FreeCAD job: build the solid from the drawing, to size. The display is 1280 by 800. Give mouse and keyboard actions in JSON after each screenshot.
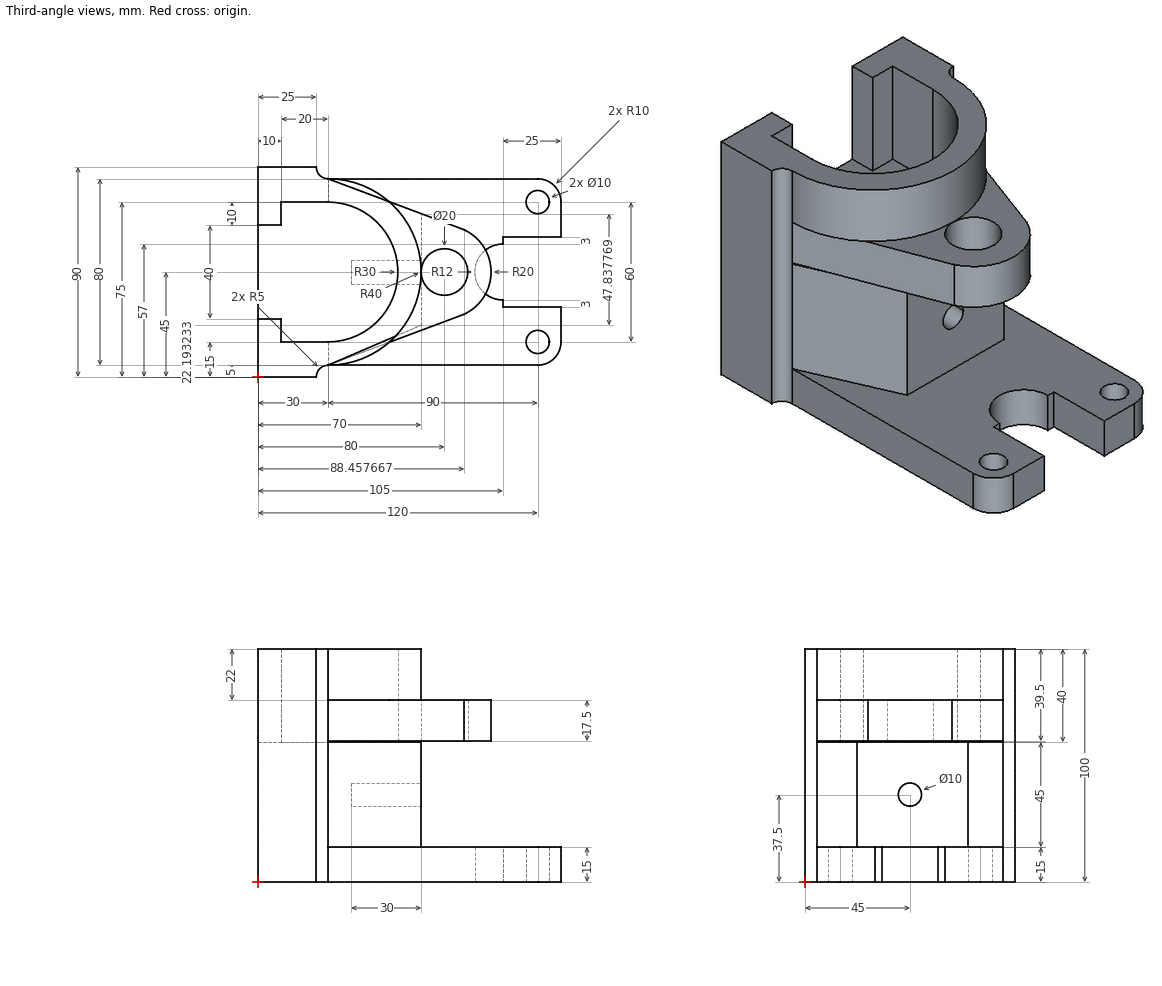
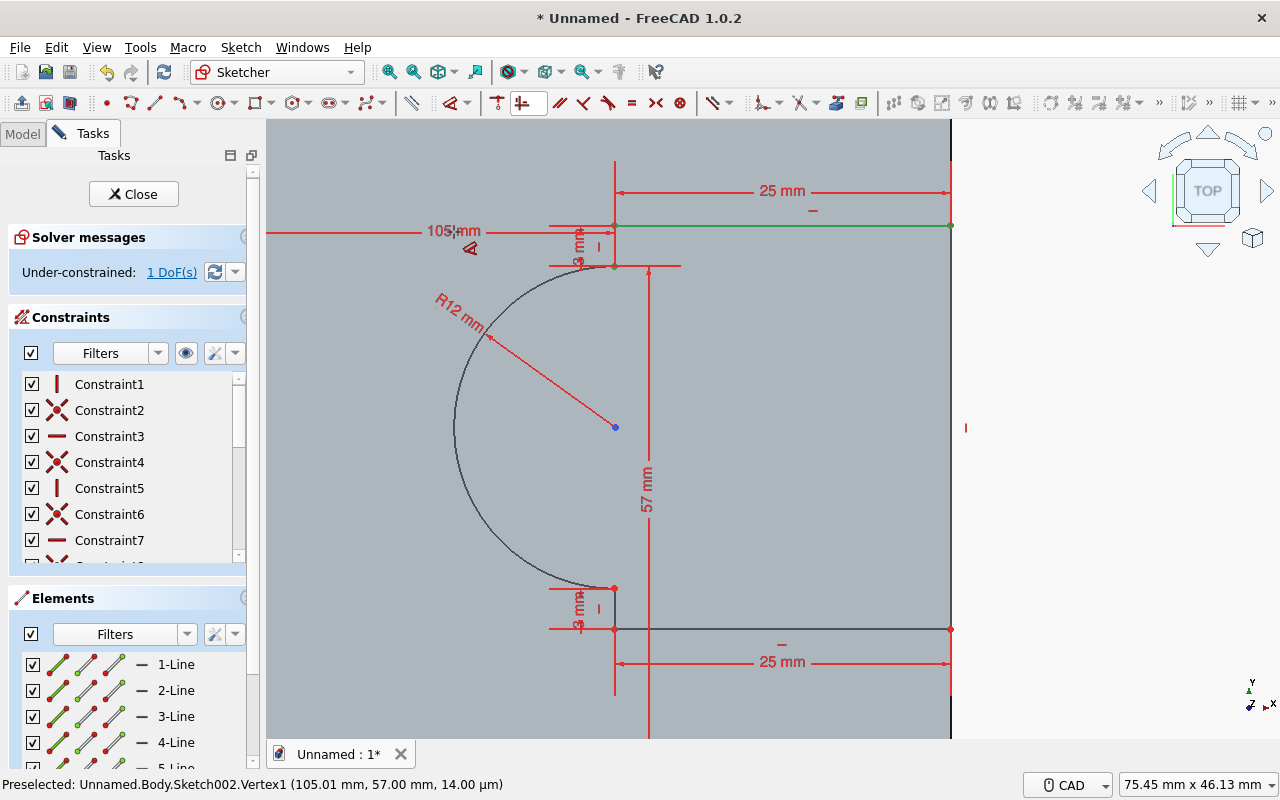
{"action": "left_click", "coordinate": [616, 427]}
{"action": "left_click", "coordinate": [381, 393]}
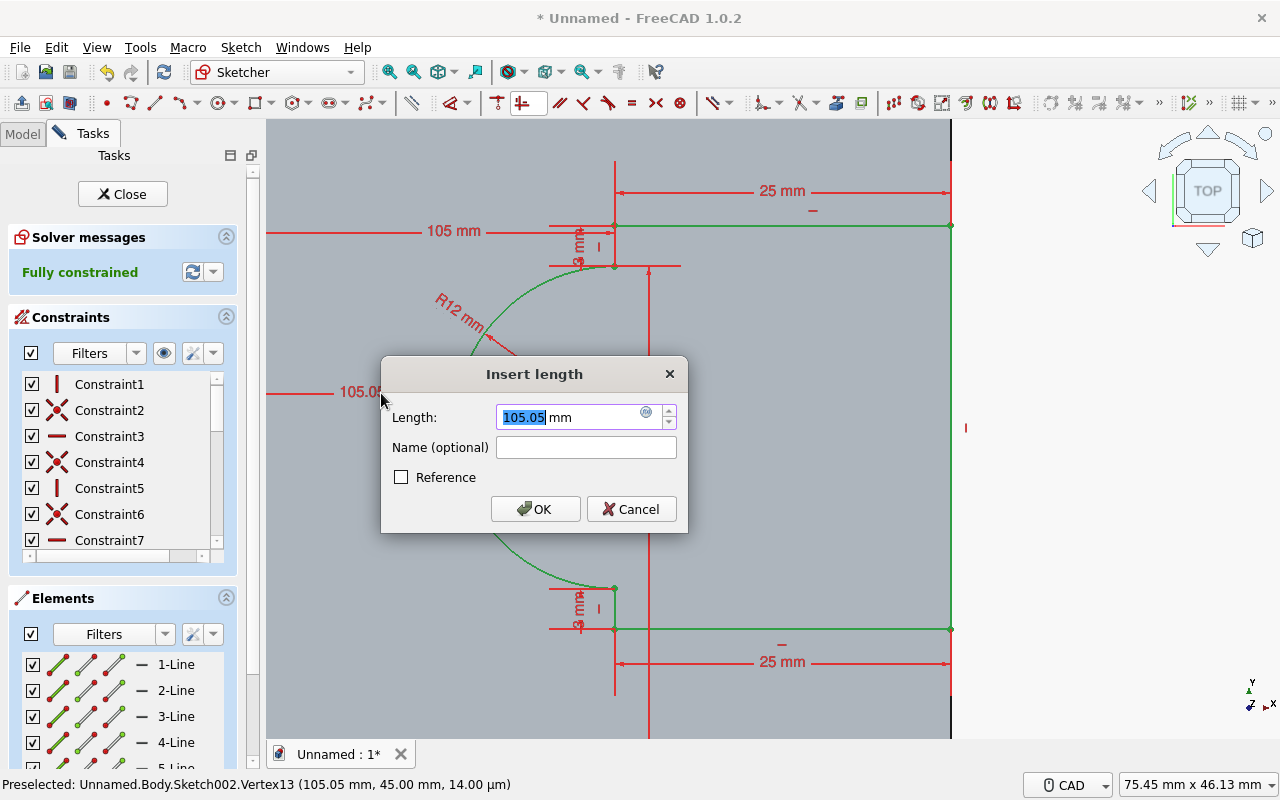
{"action": "type", "text": "105"}
{"action": "key", "text": "Return"}
{"action": "key", "text": "Escape"}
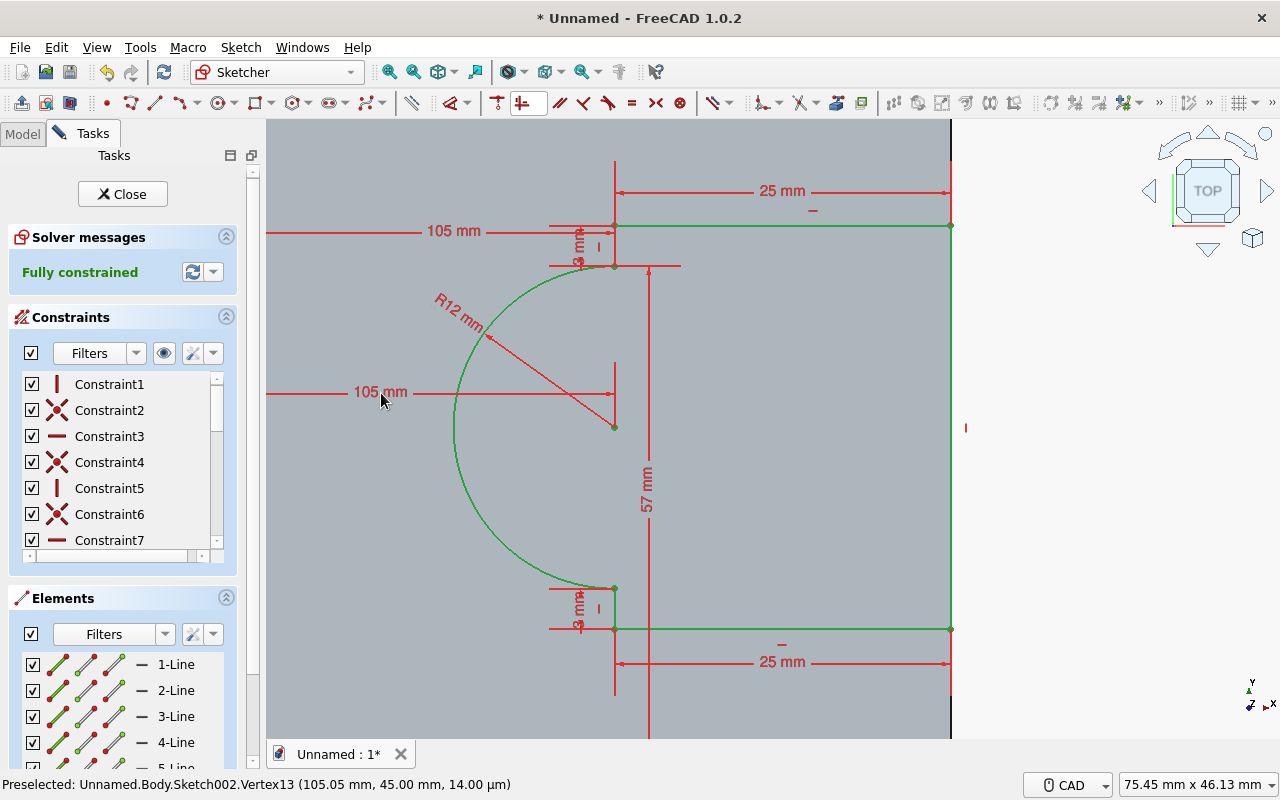
{"action": "left_click", "coordinate": [123, 194]}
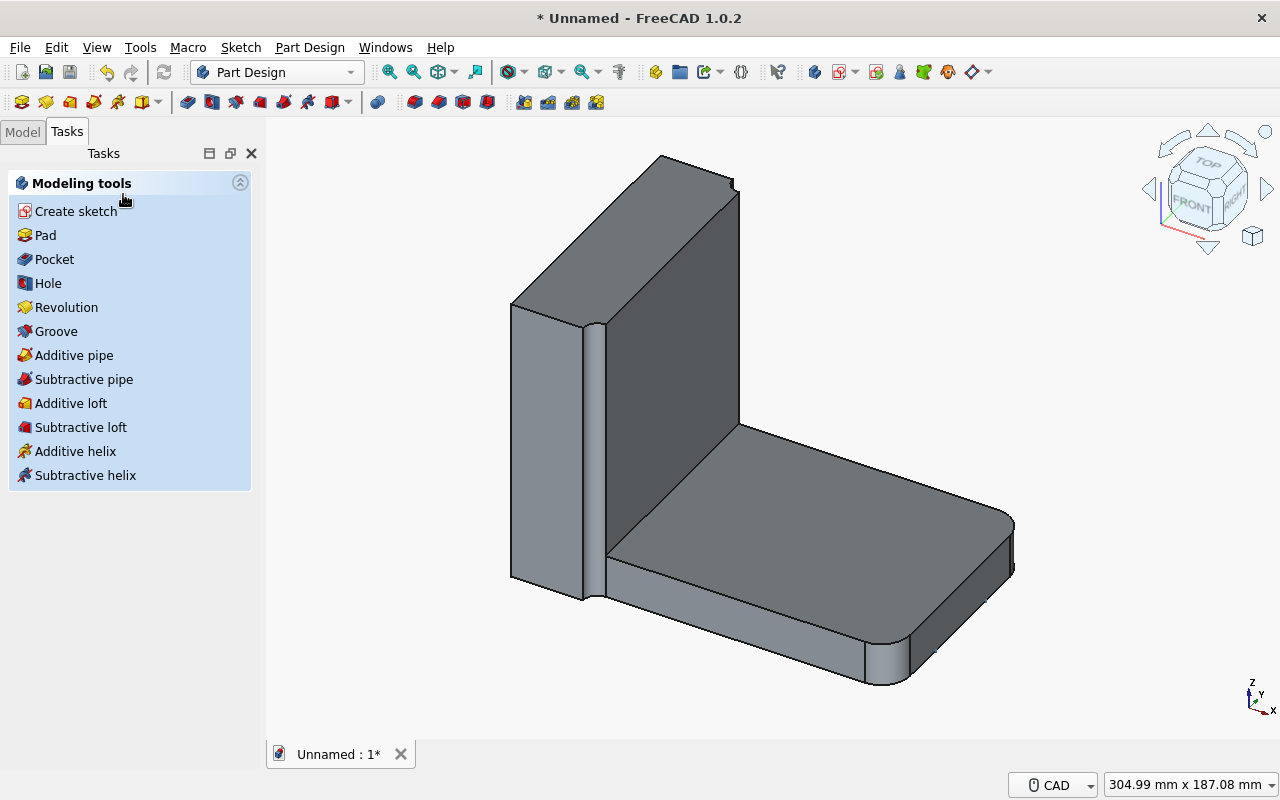
{"action": "left_click", "coordinate": [188, 102]}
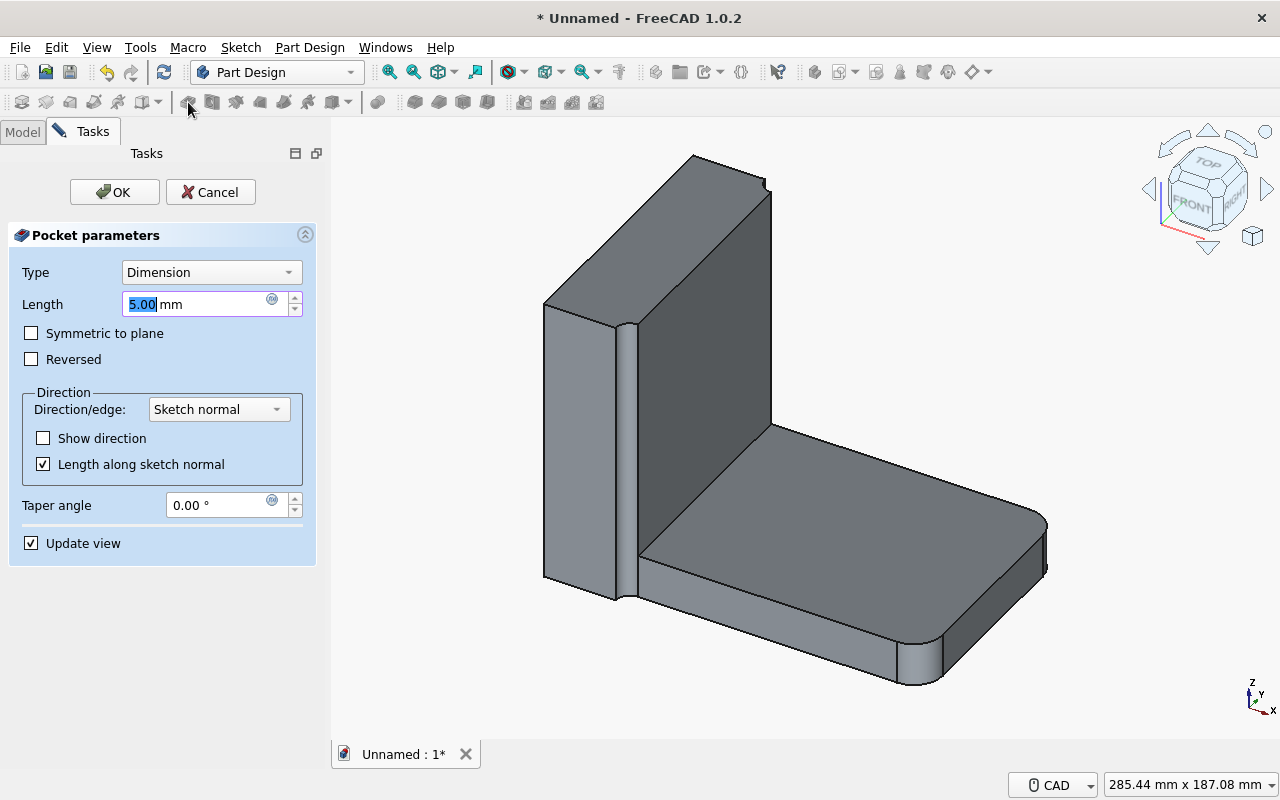
{"action": "type", "text": "15"}
{"action": "key", "text": "Tab"}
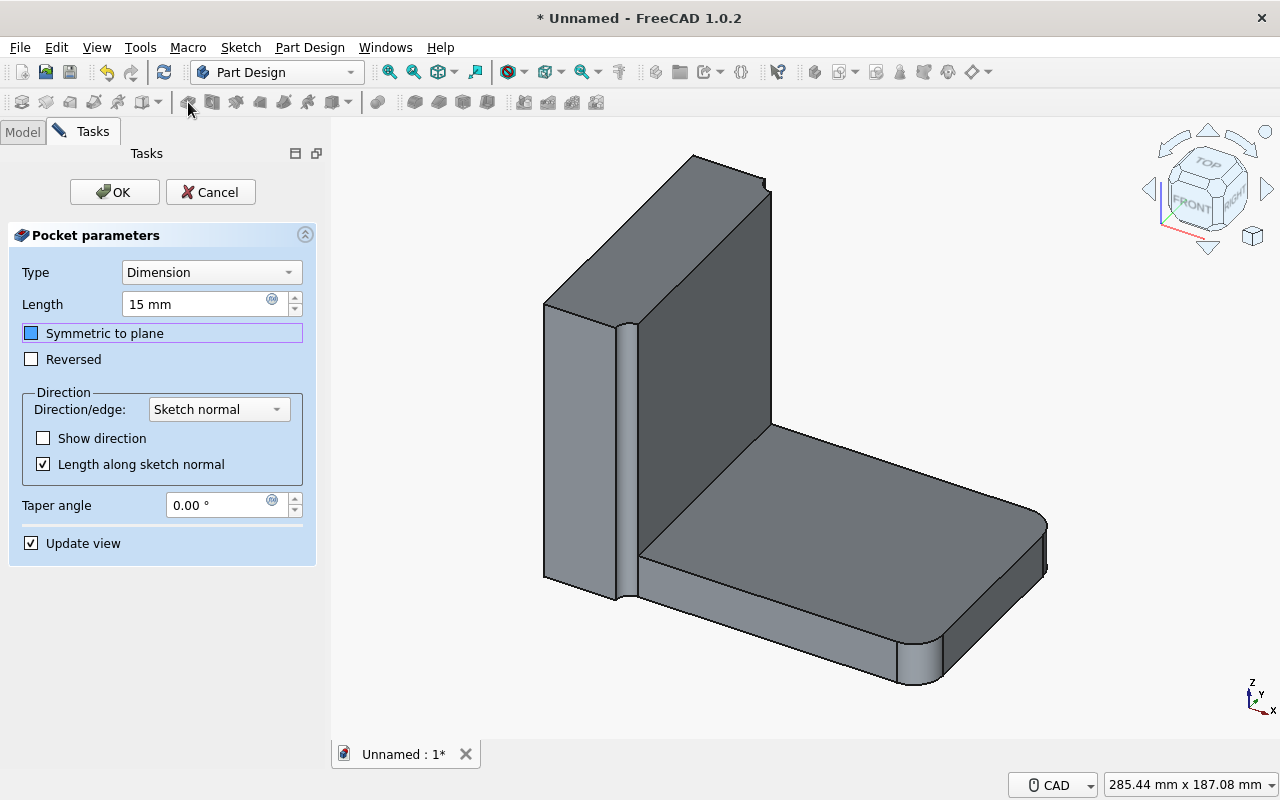
{"action": "left_click", "coordinate": [30, 359]}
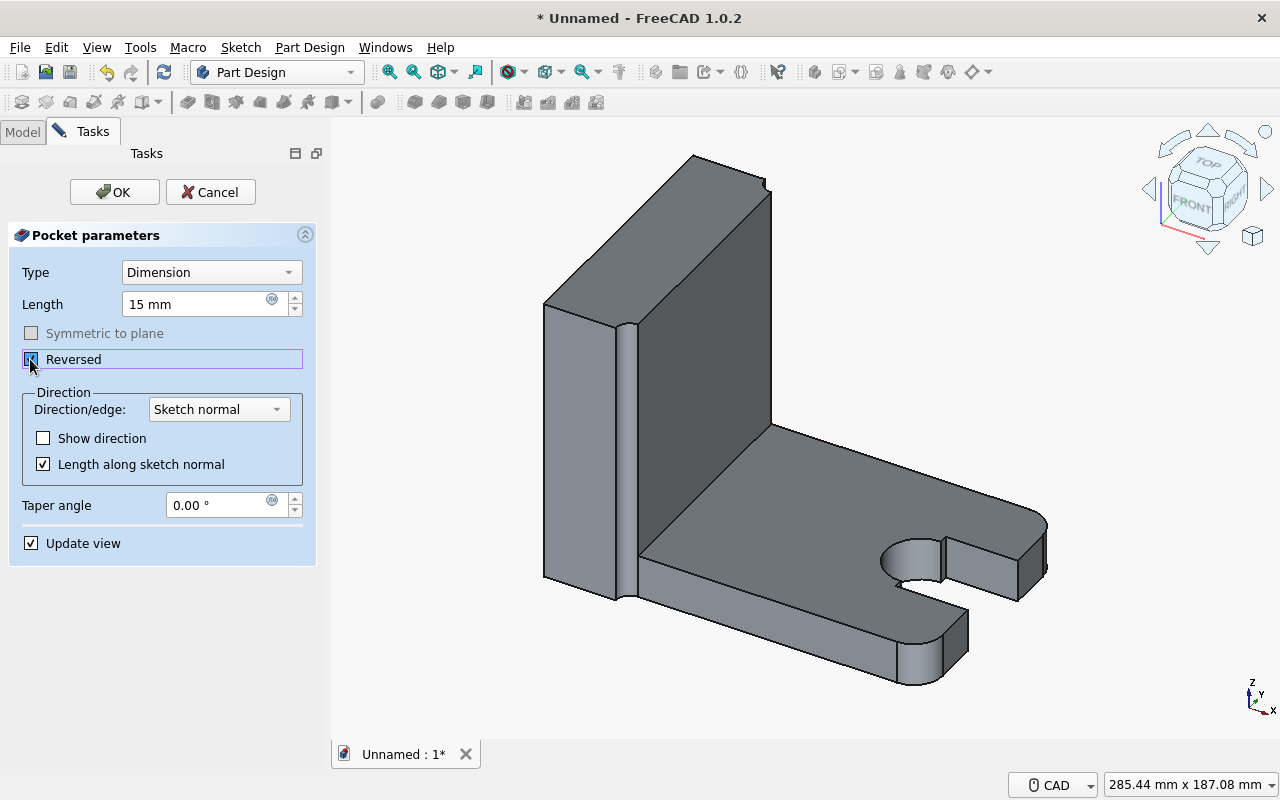
{"action": "left_click", "coordinate": [115, 192]}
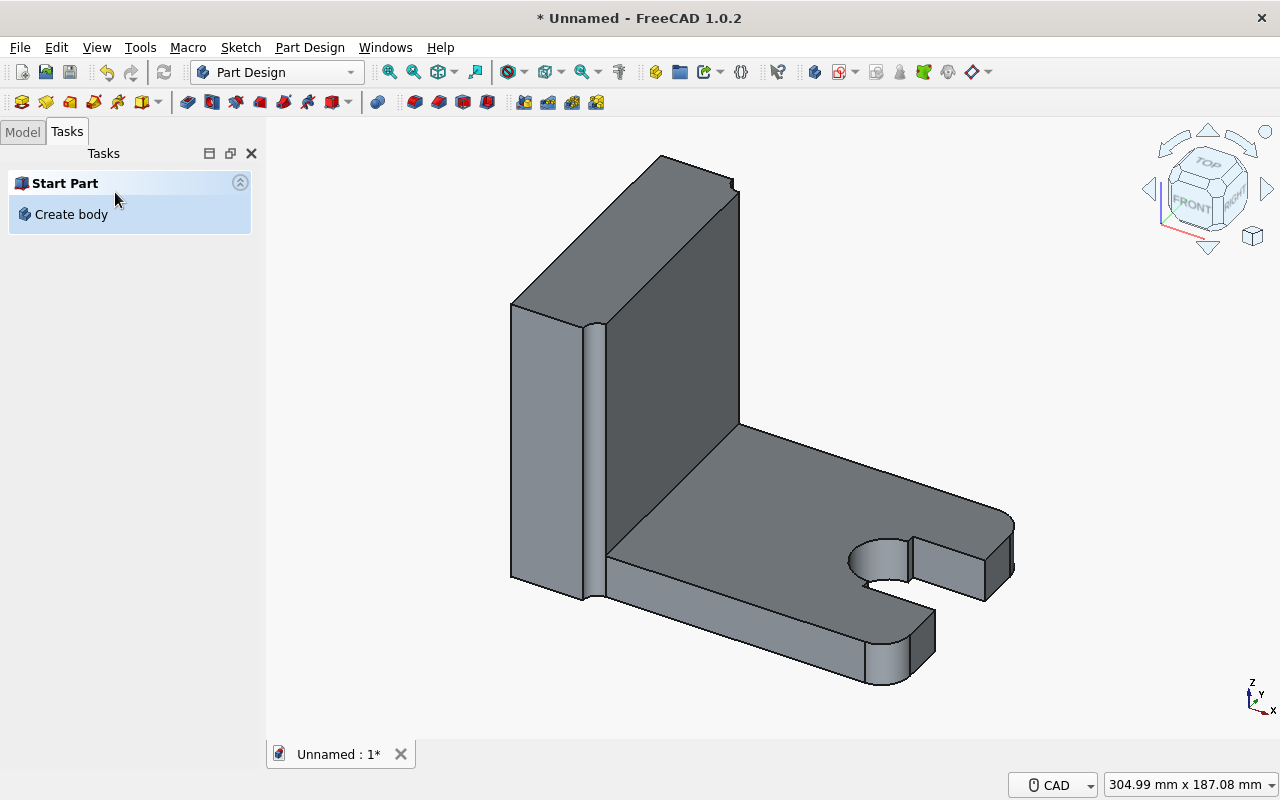
{"action": "left_click", "coordinate": [794, 504]}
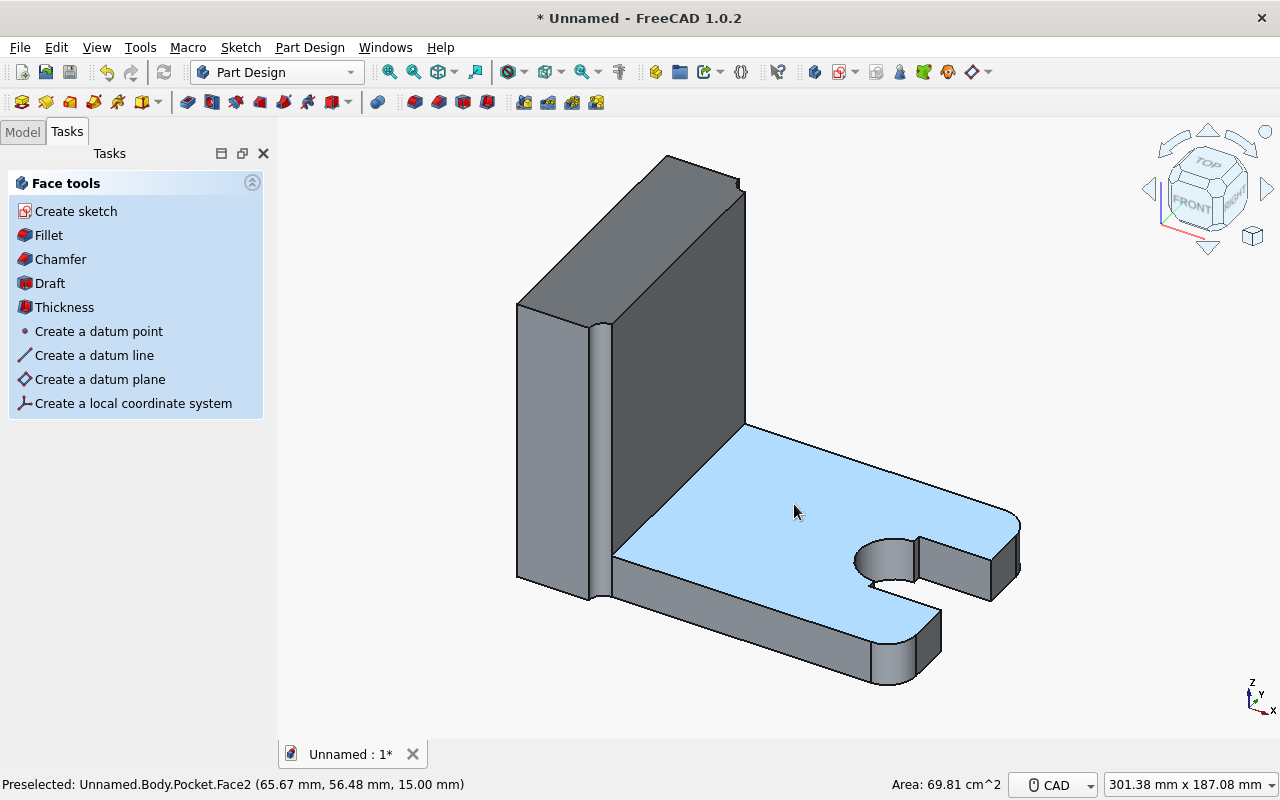
{"action": "left_click", "coordinate": [840, 72]}